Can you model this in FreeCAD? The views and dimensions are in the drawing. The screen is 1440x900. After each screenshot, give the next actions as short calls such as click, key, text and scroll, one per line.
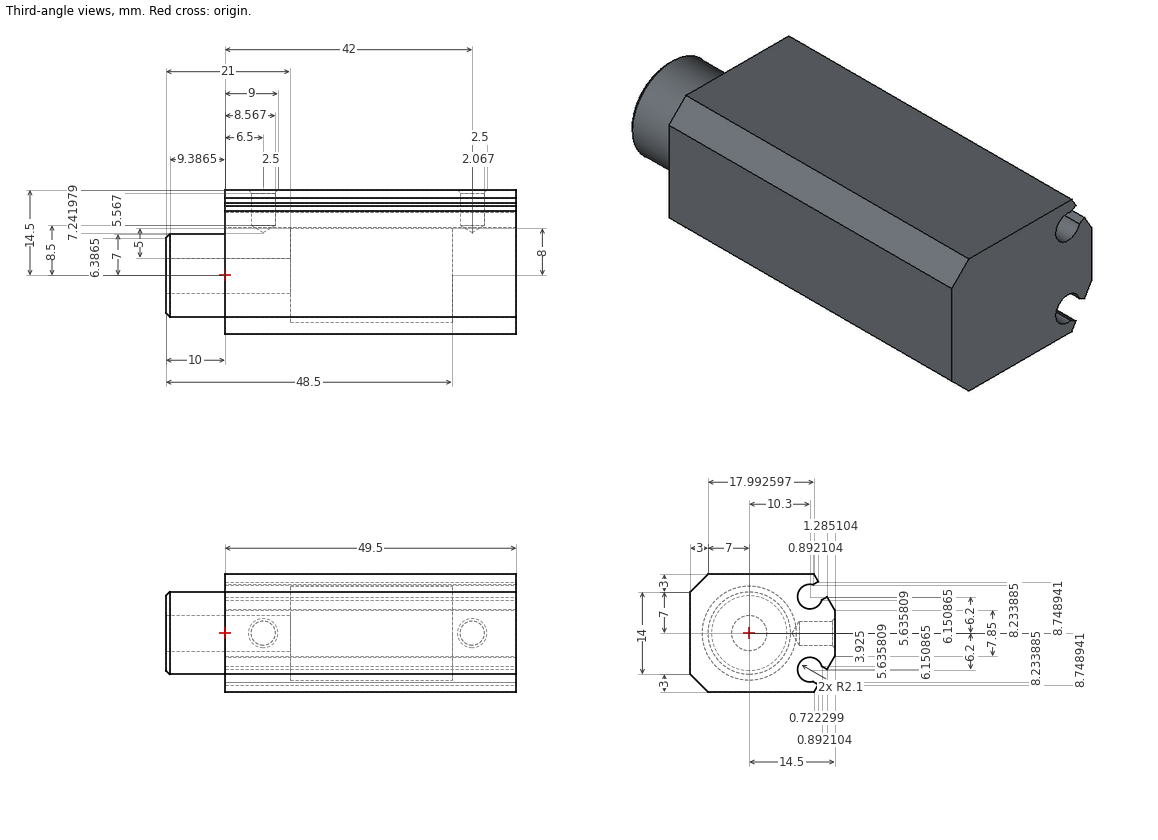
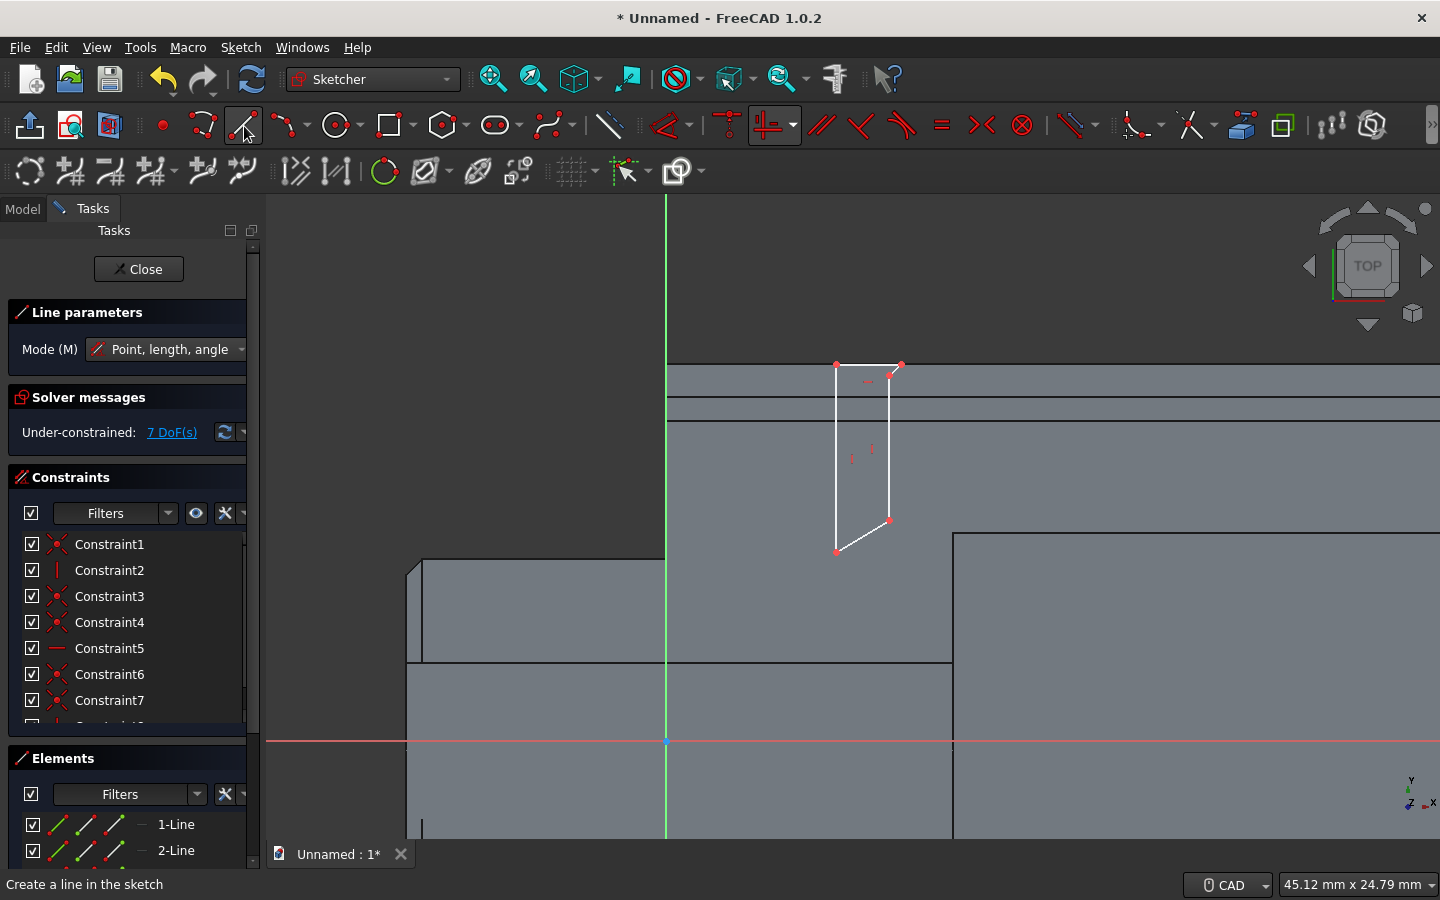
click(836, 345)
click(836, 289)
key(Escape)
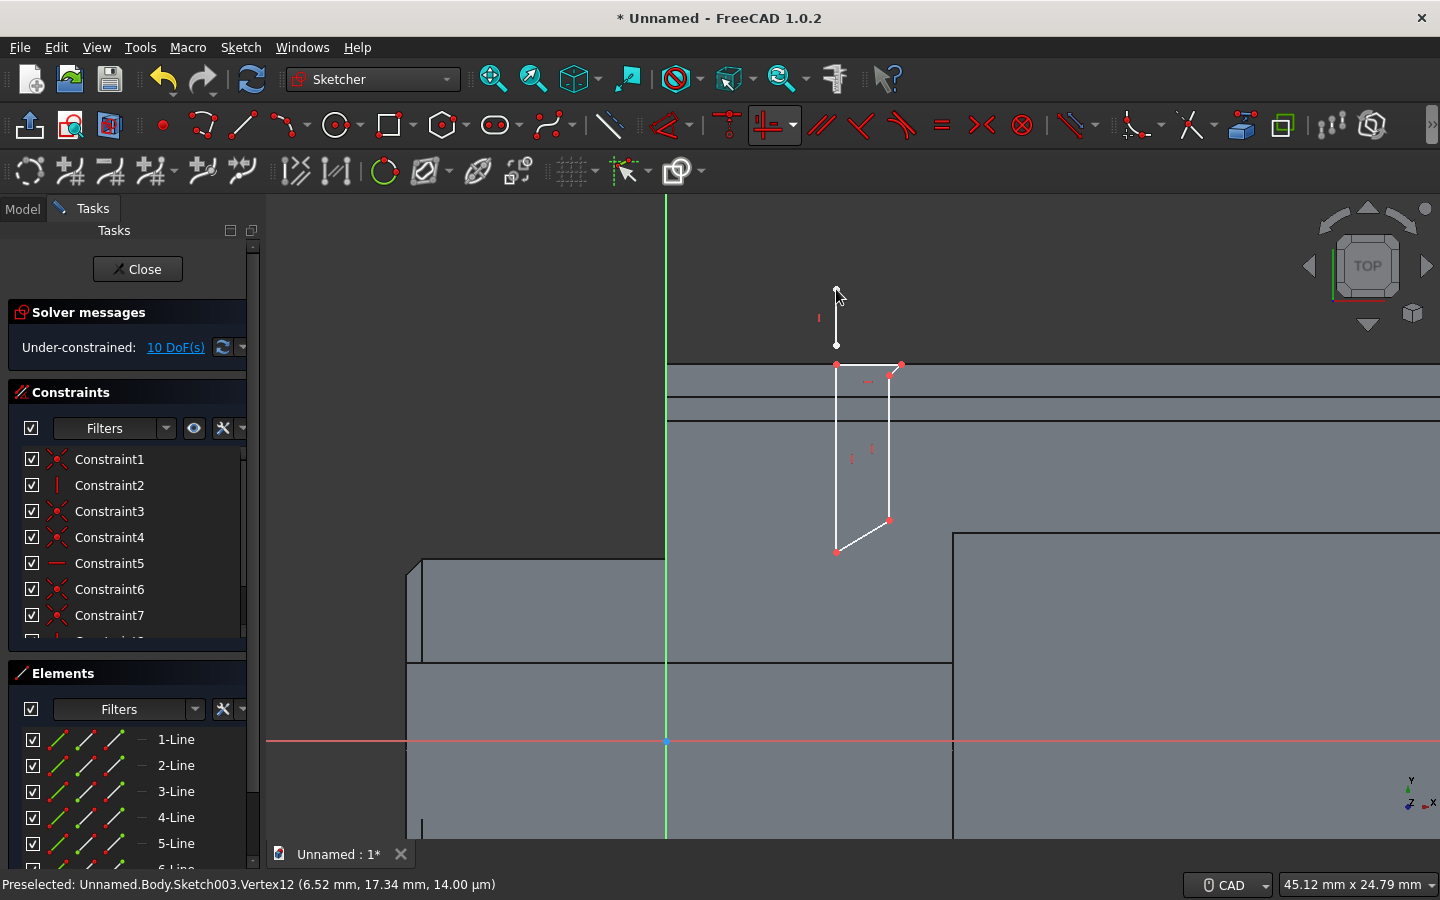
click(836, 329)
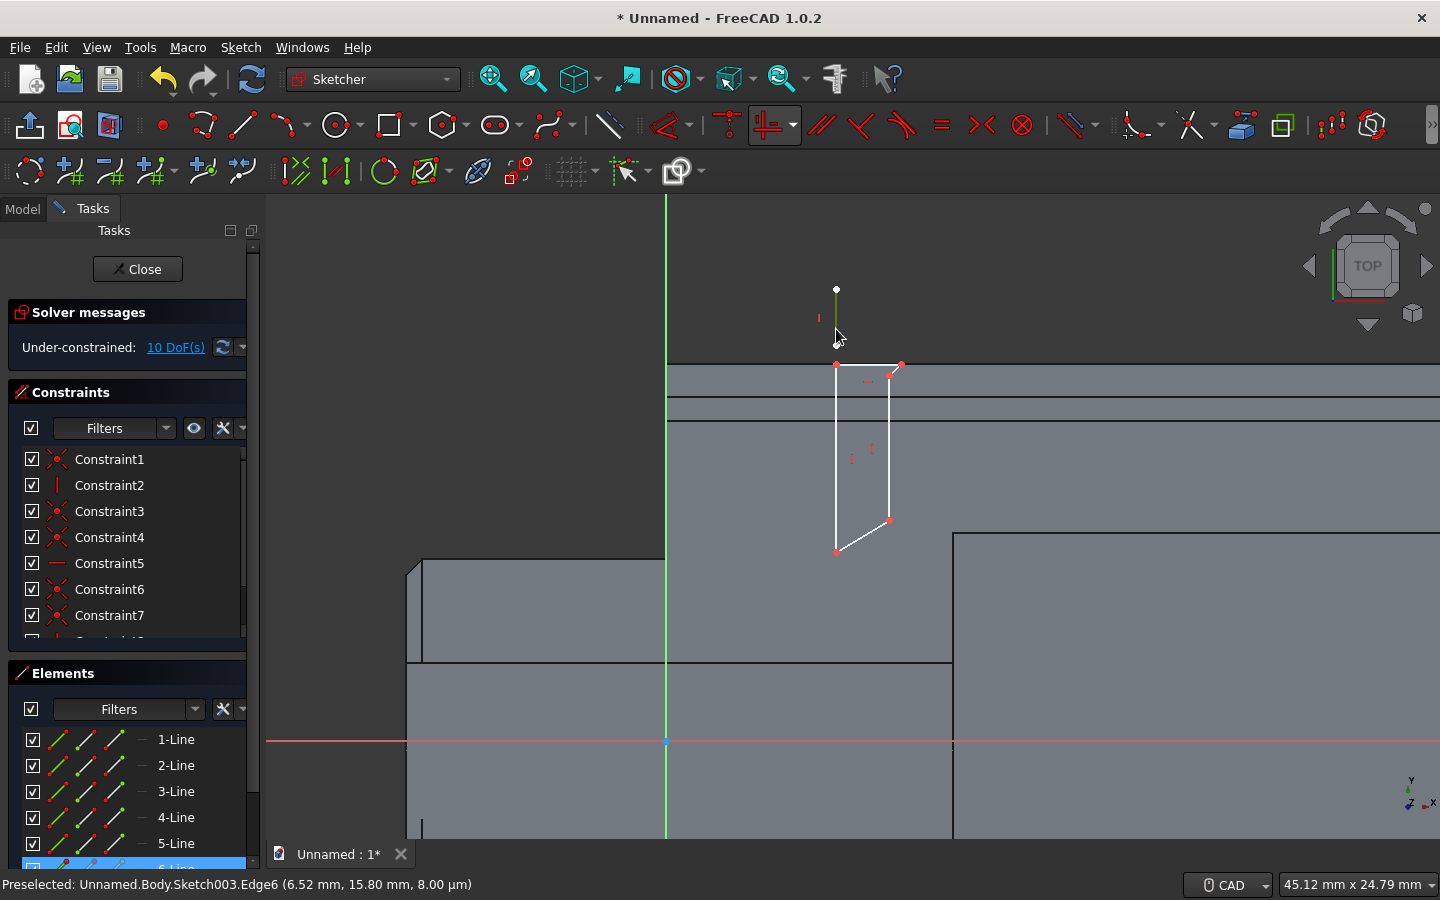
click(610, 126)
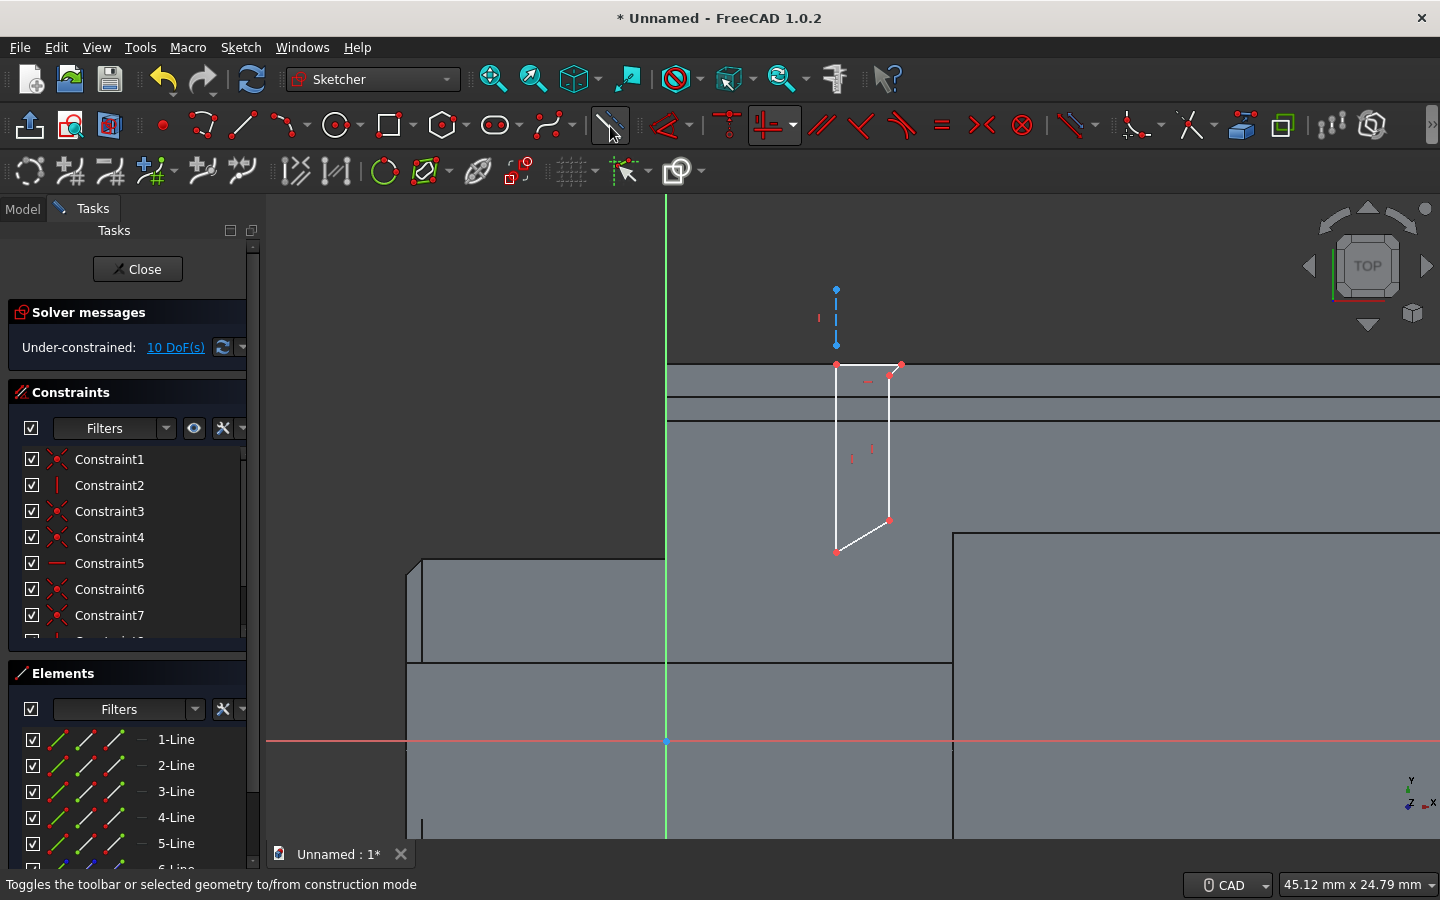
click(664, 126)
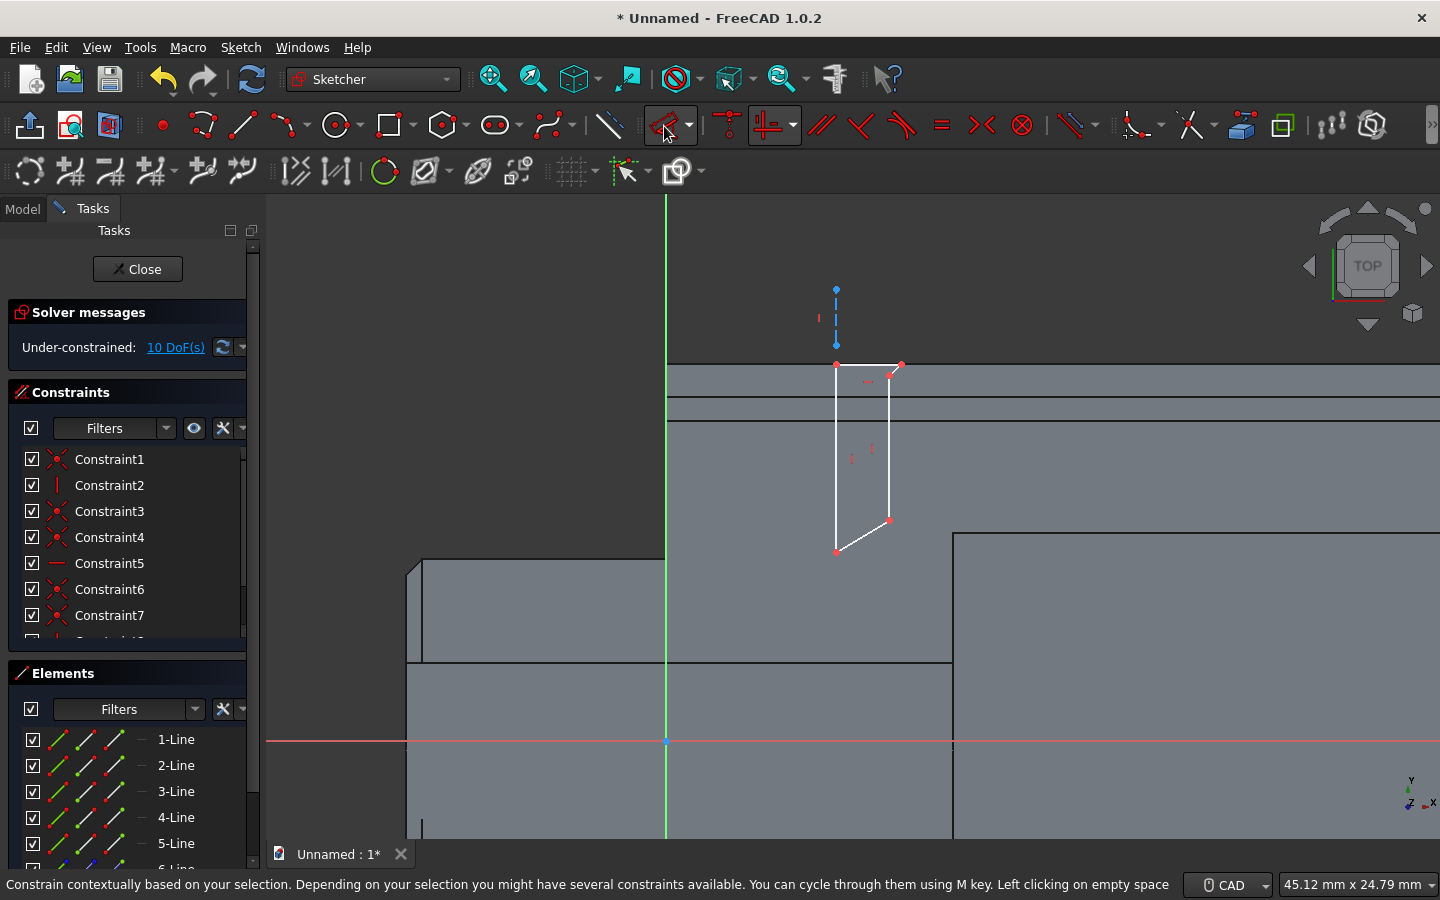
click(901, 365)
click(784, 775)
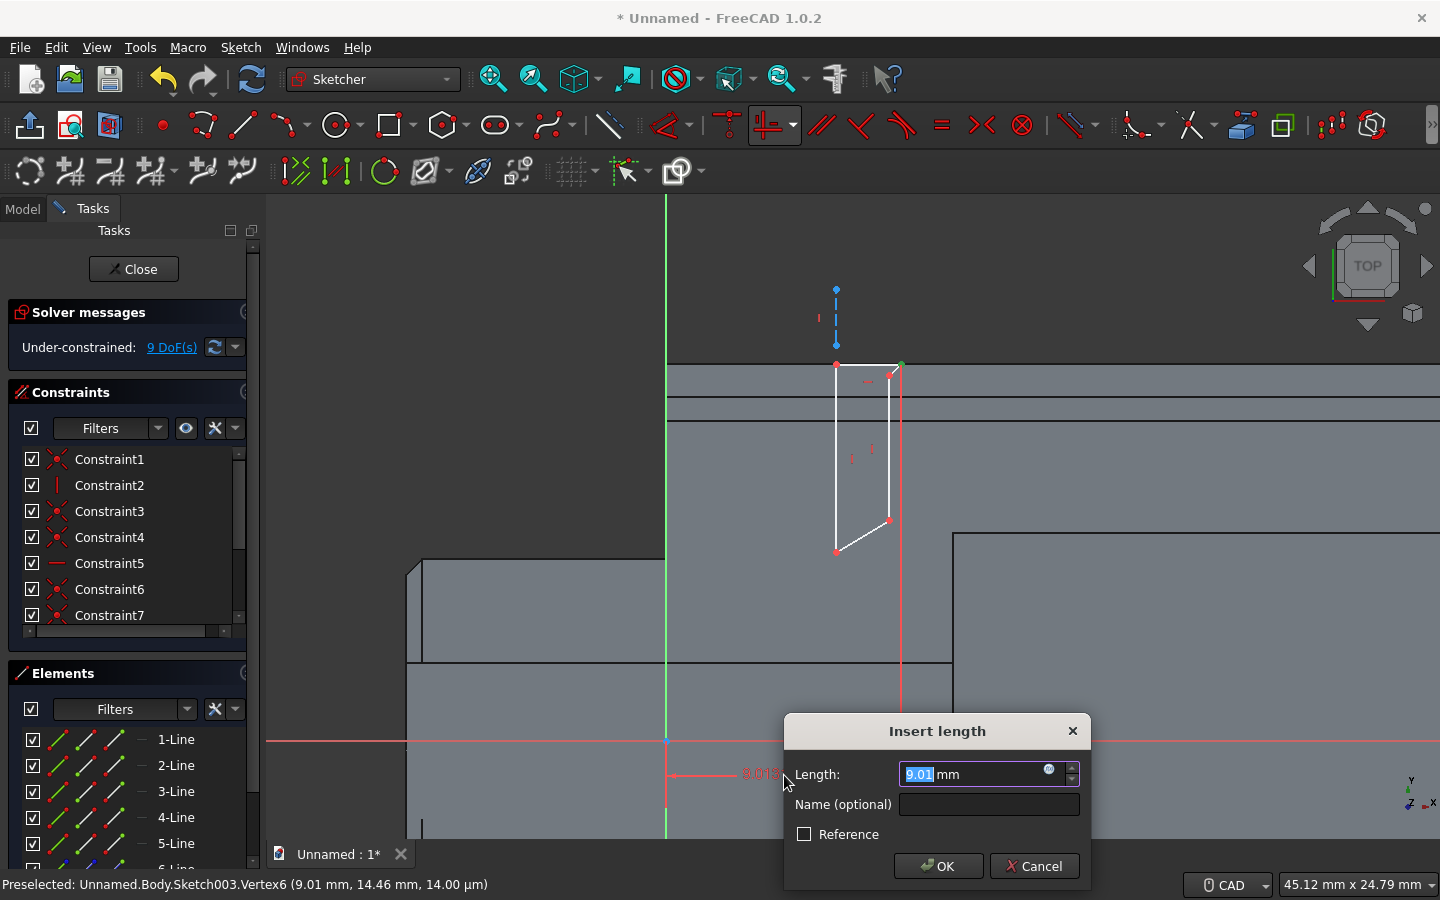
text(9)
key(Return)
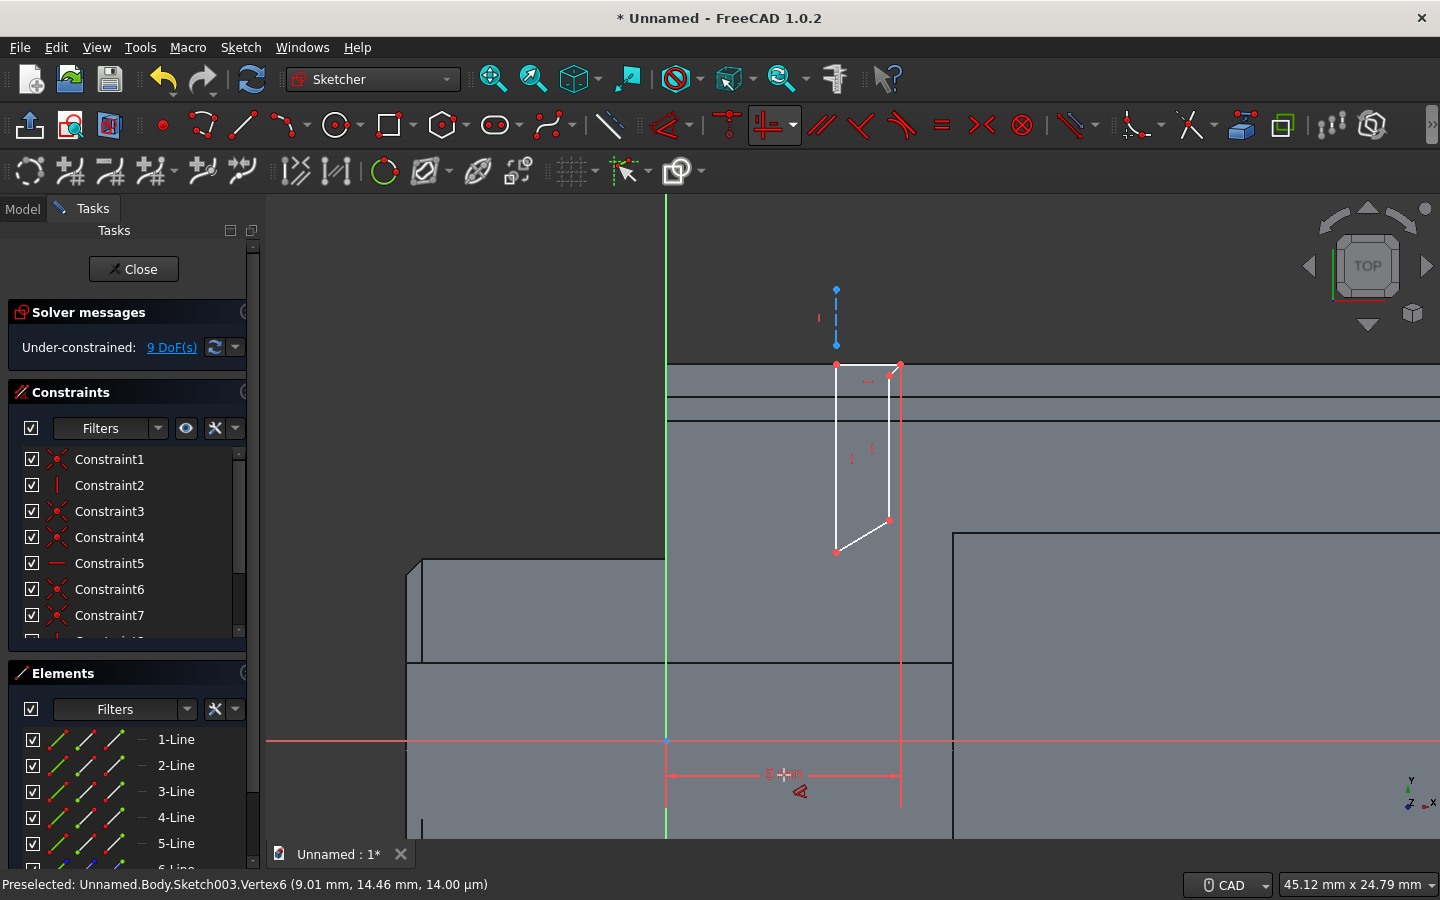
click(881, 365)
click(868, 331)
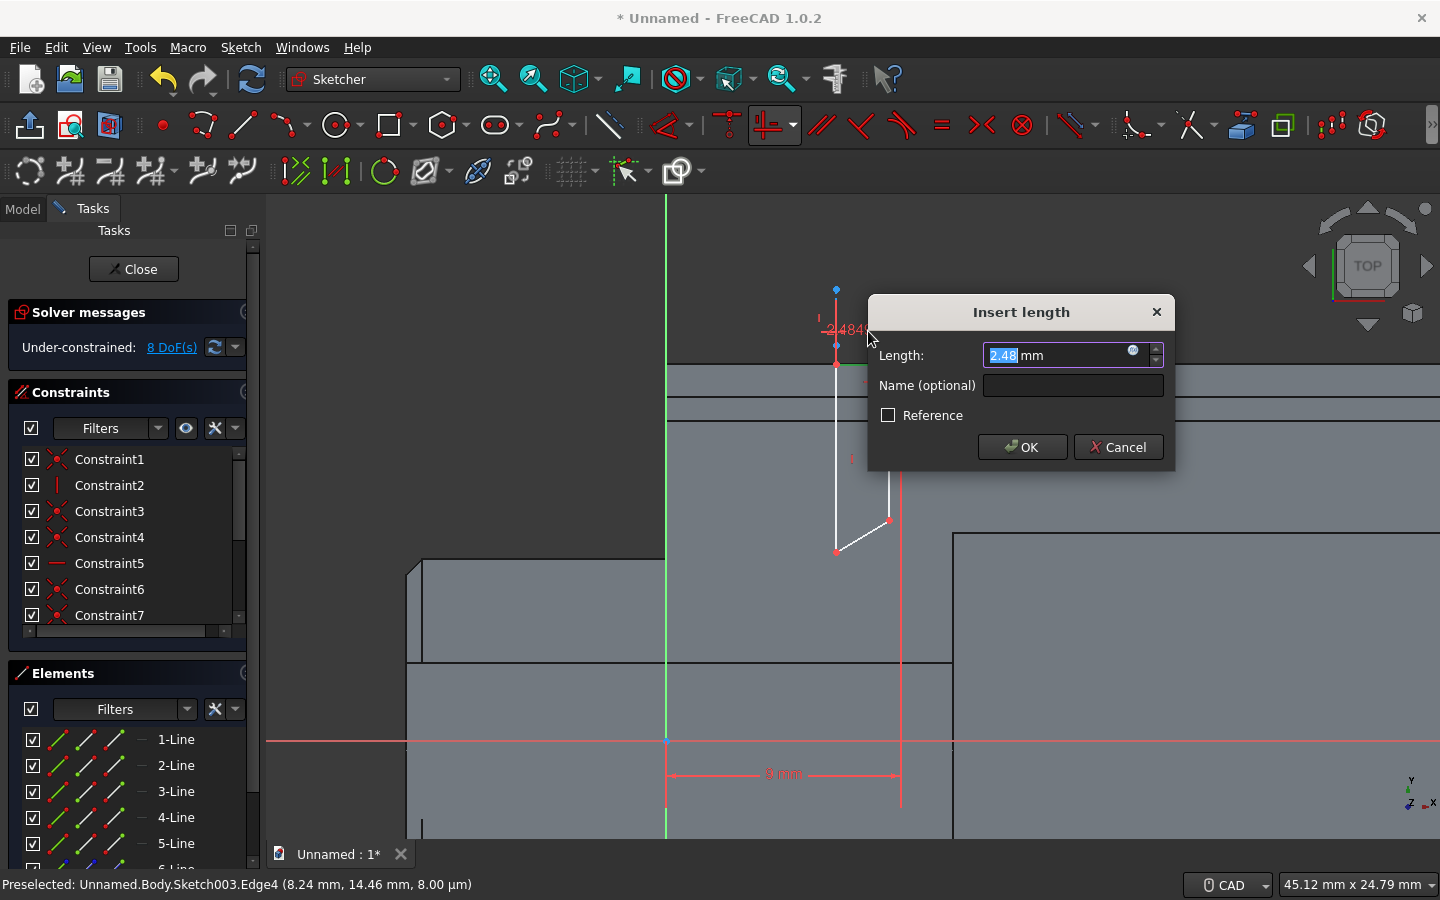
text(2.5)
key(Return)